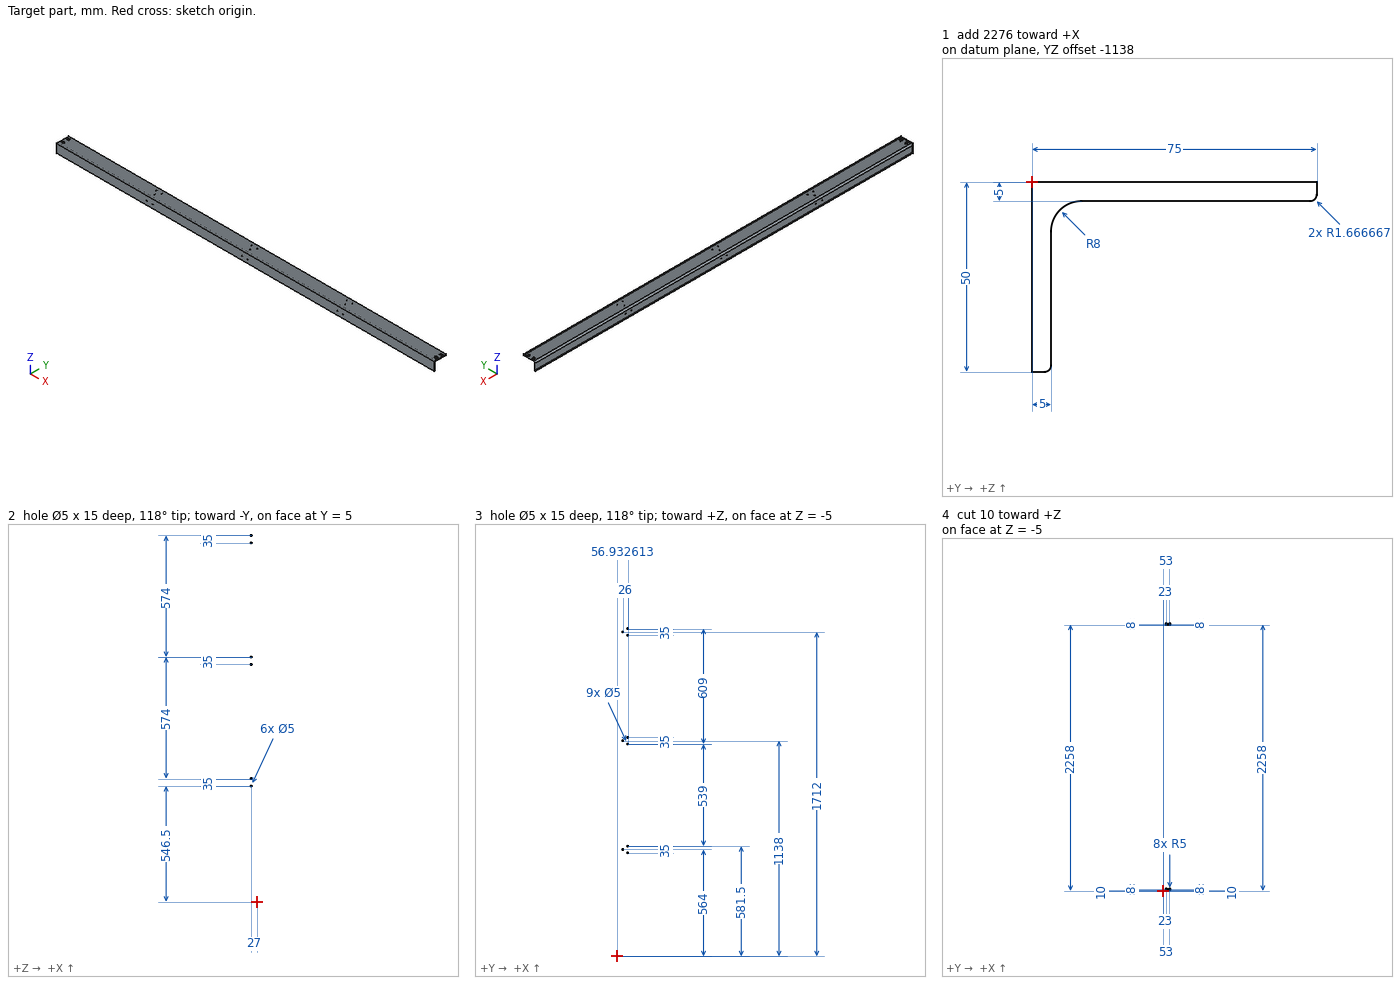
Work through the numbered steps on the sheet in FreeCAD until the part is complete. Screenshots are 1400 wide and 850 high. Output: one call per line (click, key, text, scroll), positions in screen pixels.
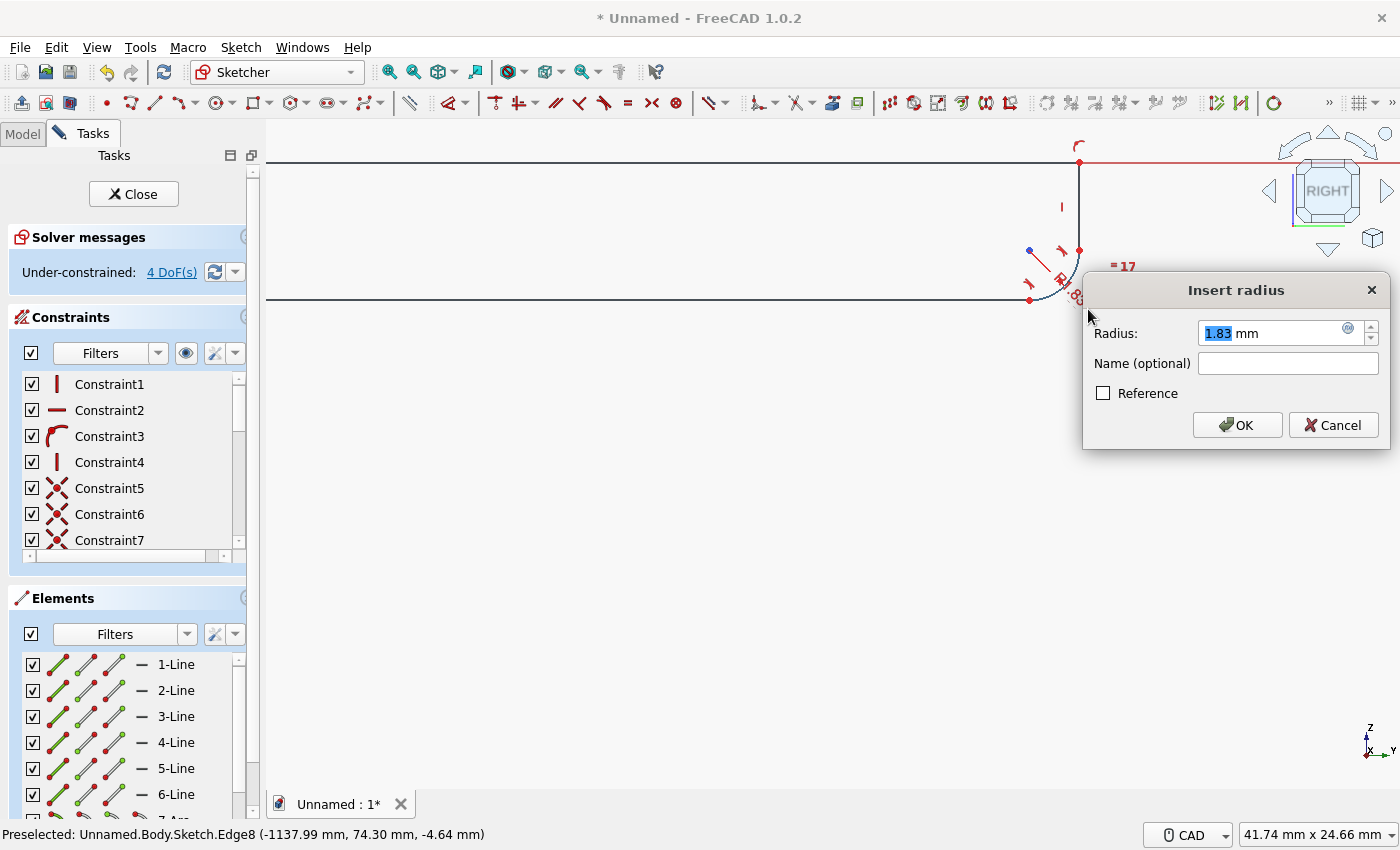
text(1.666667)
key(Return)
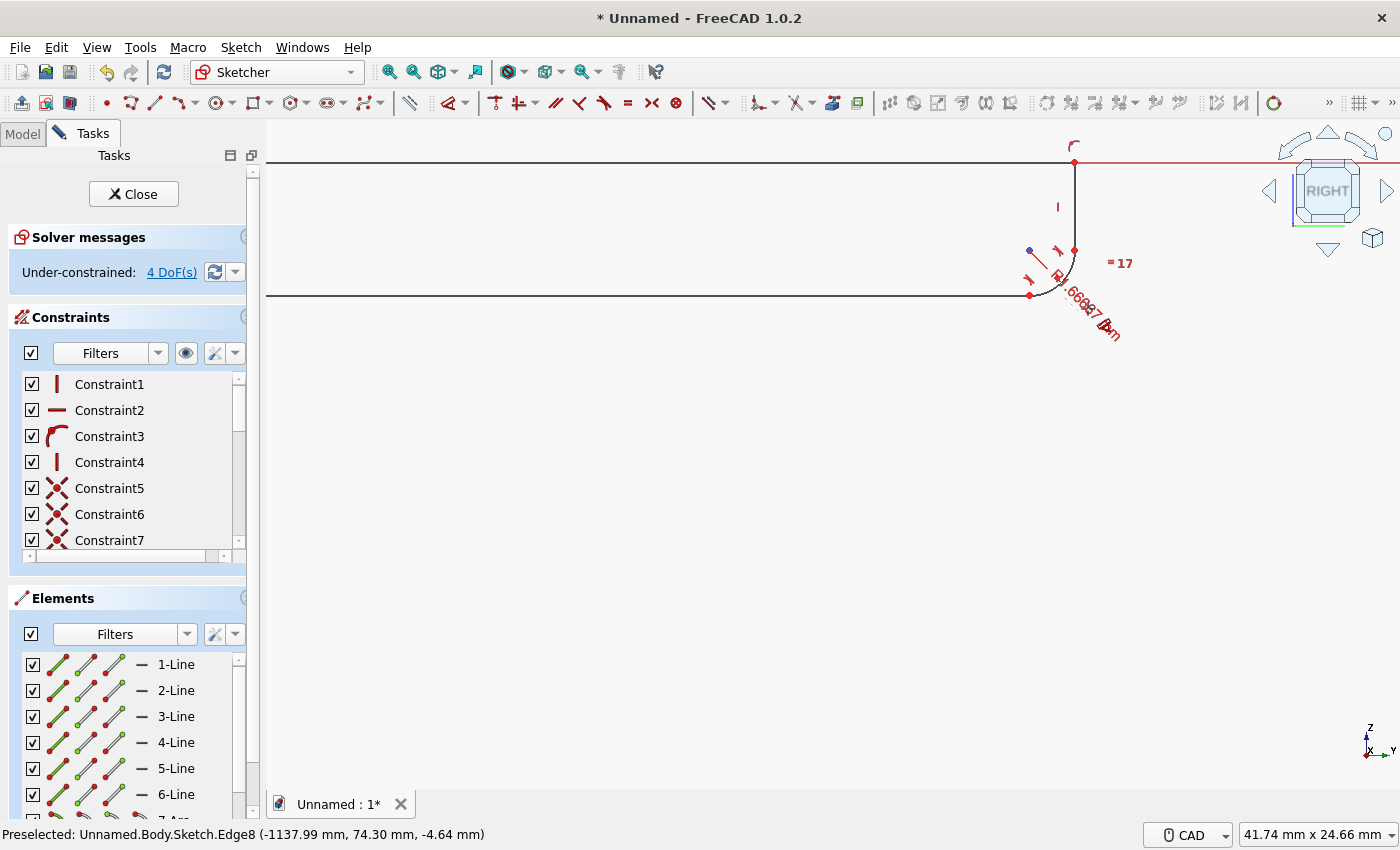
click(465, 163)
click(684, 197)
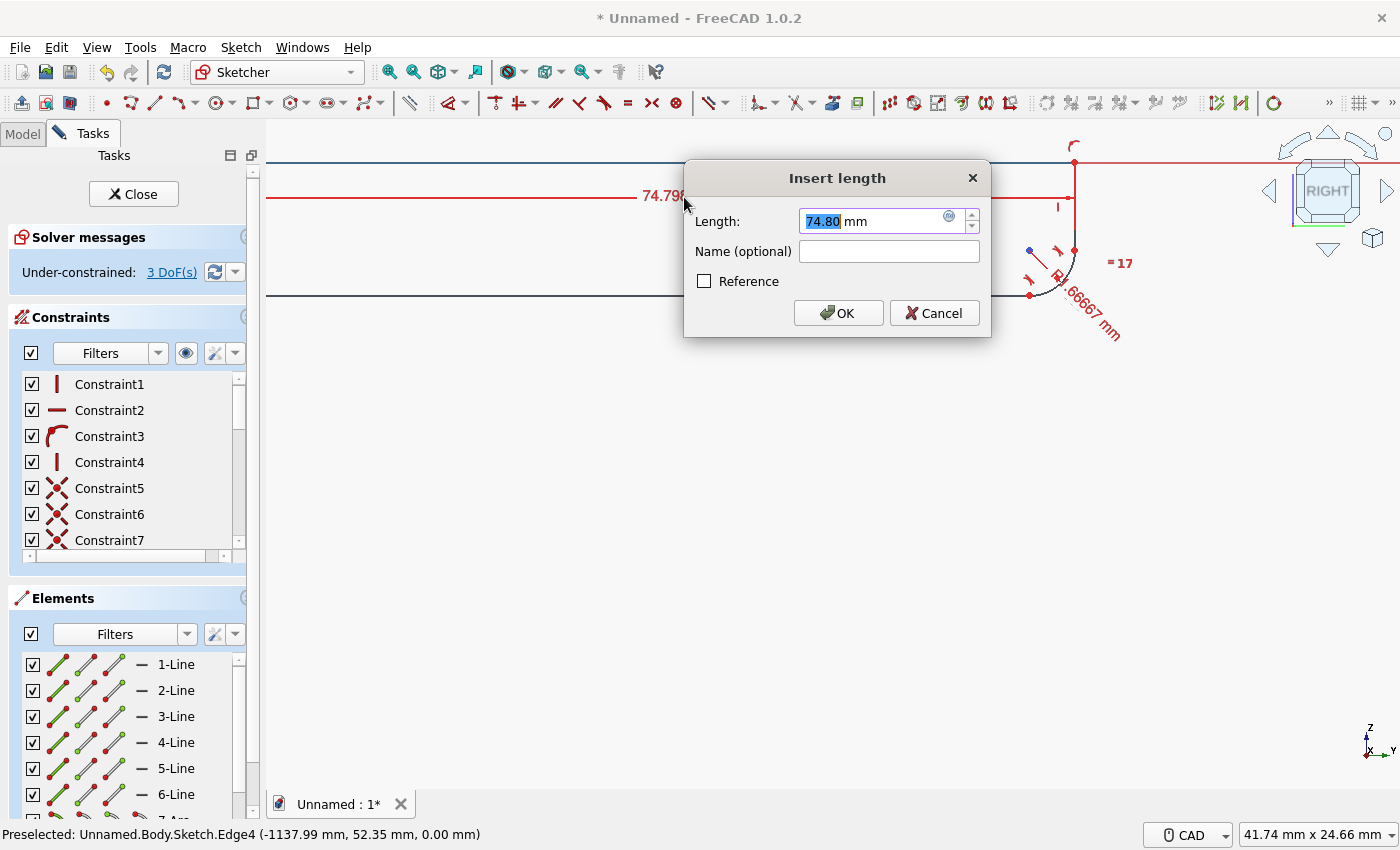
text(75)
key(Return)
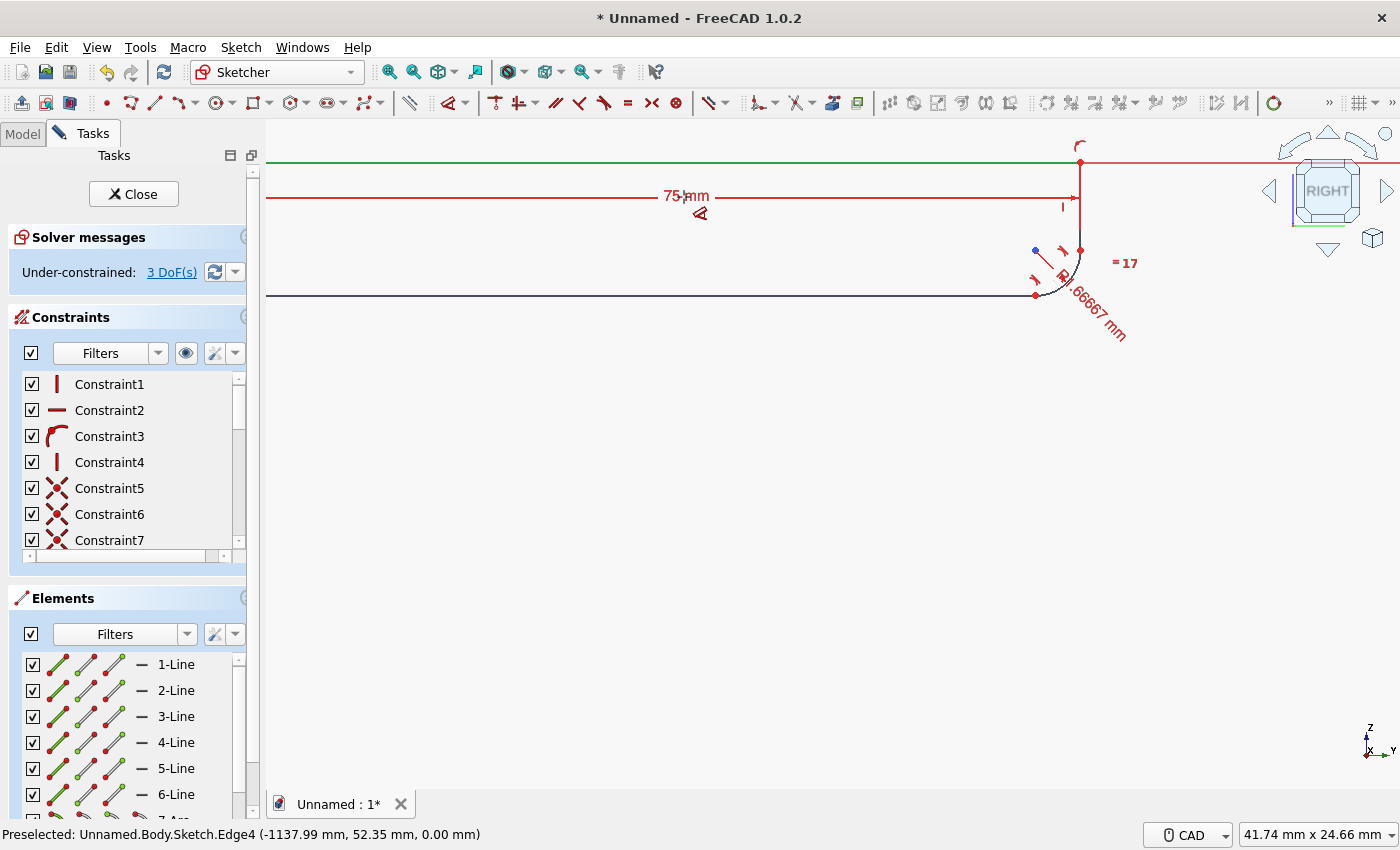
scroll(1067, 287, down, 6)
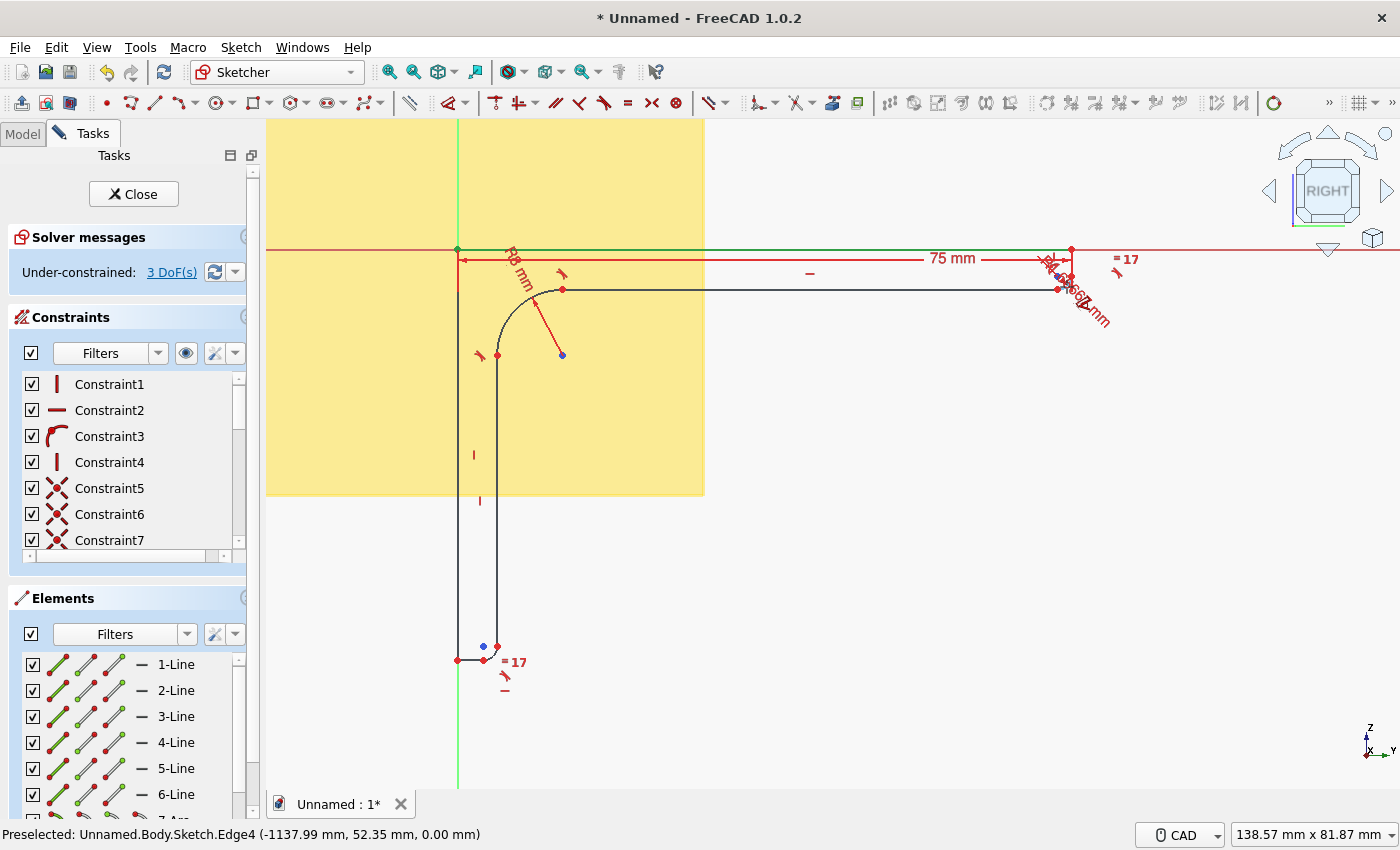
click(458, 373)
click(424, 455)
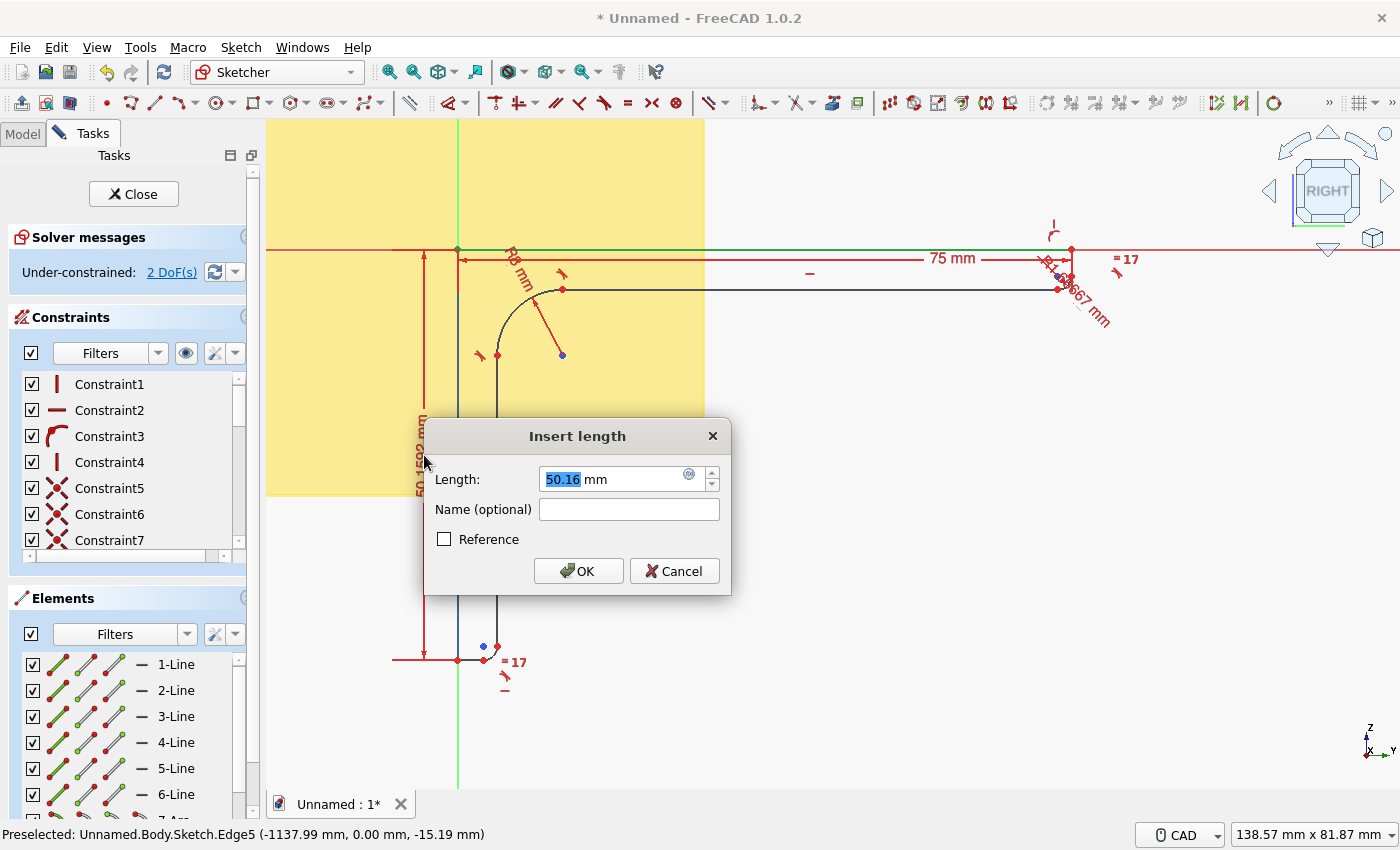
text(50)
key(Return)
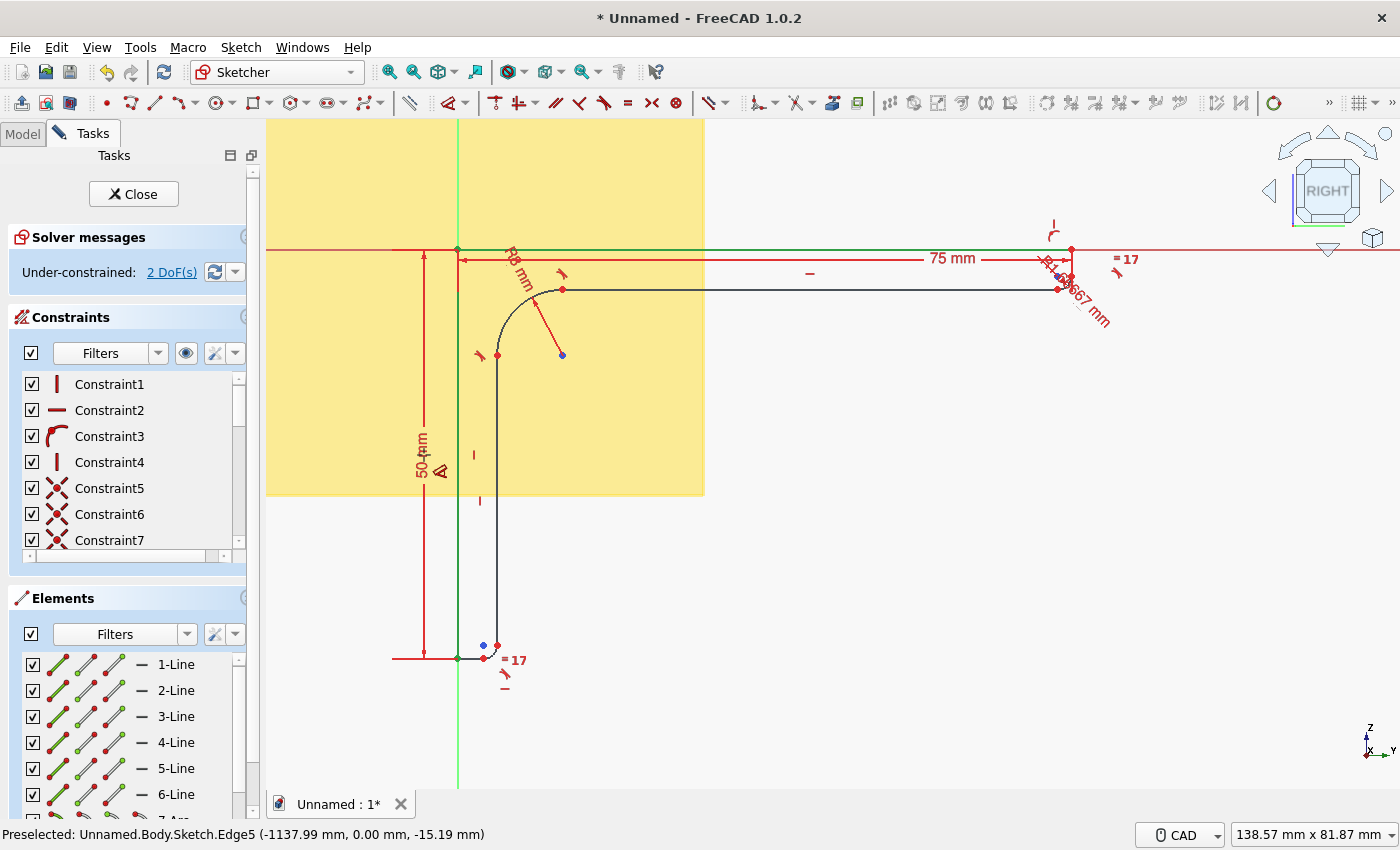
click(497, 645)
click(477, 216)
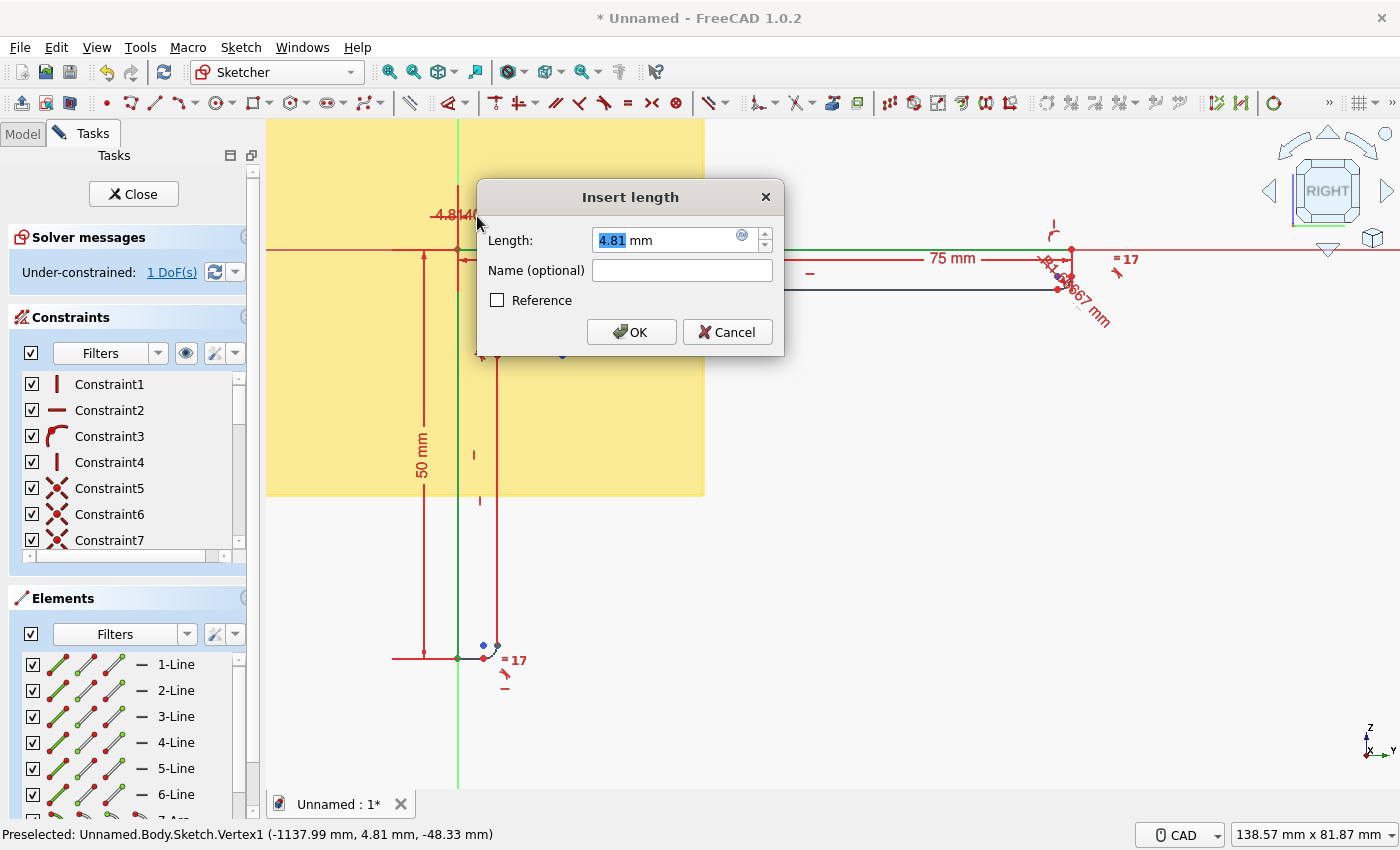
text(5)
key(Return)